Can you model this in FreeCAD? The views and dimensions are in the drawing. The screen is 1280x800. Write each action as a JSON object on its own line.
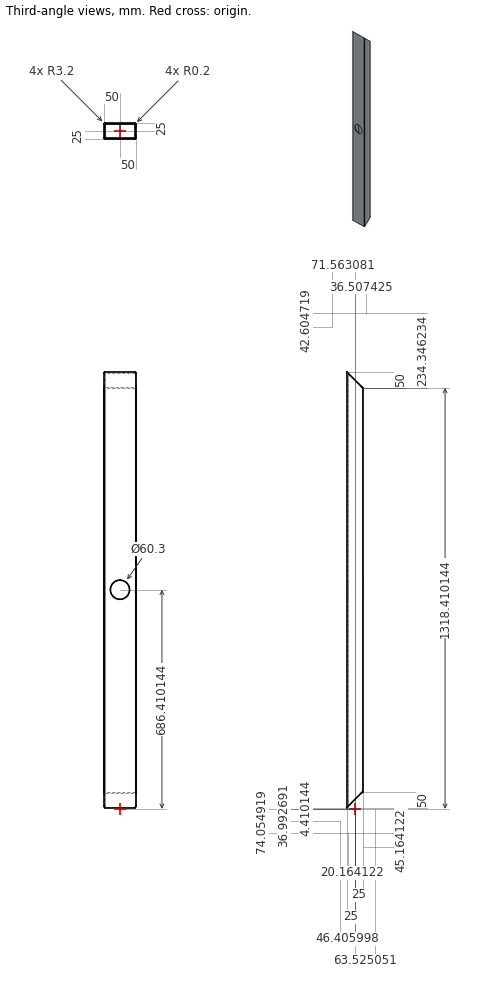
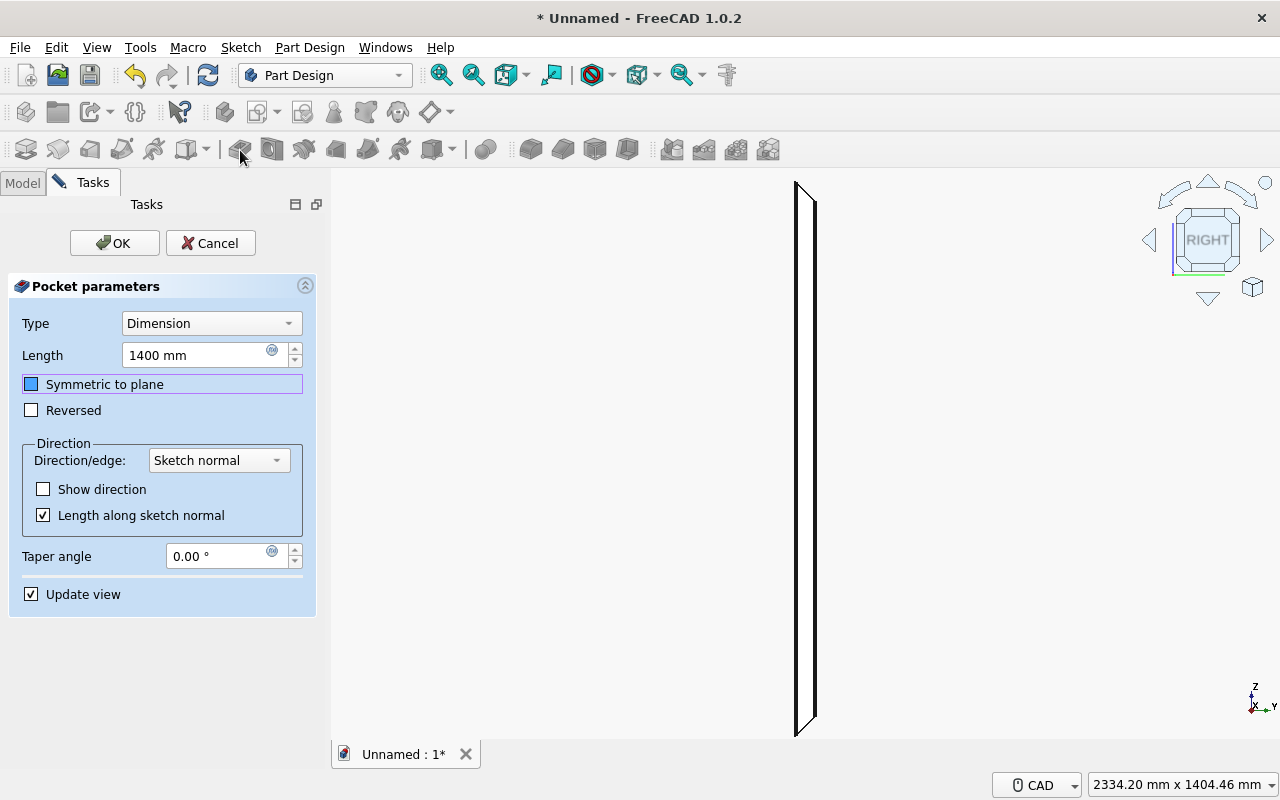
{"action": "left_click", "coordinate": [115, 243]}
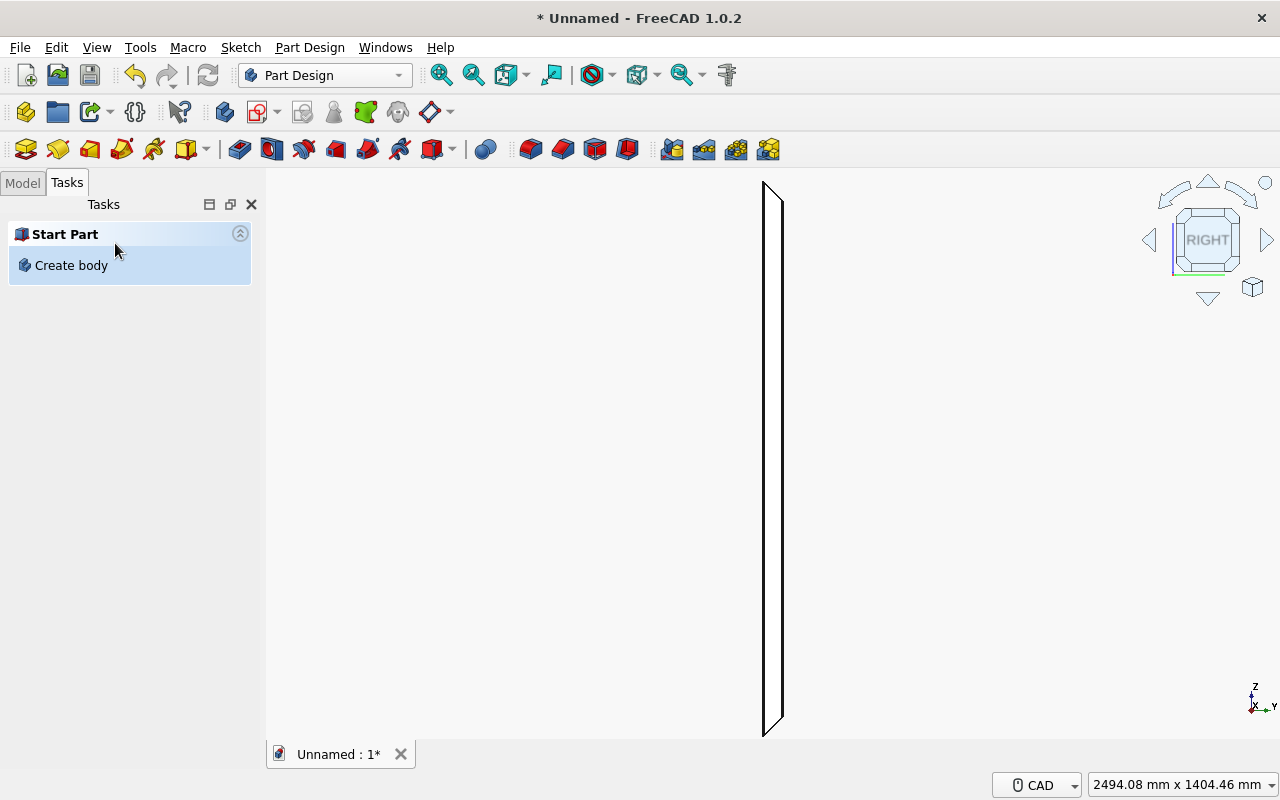
{"action": "key", "text": "4"}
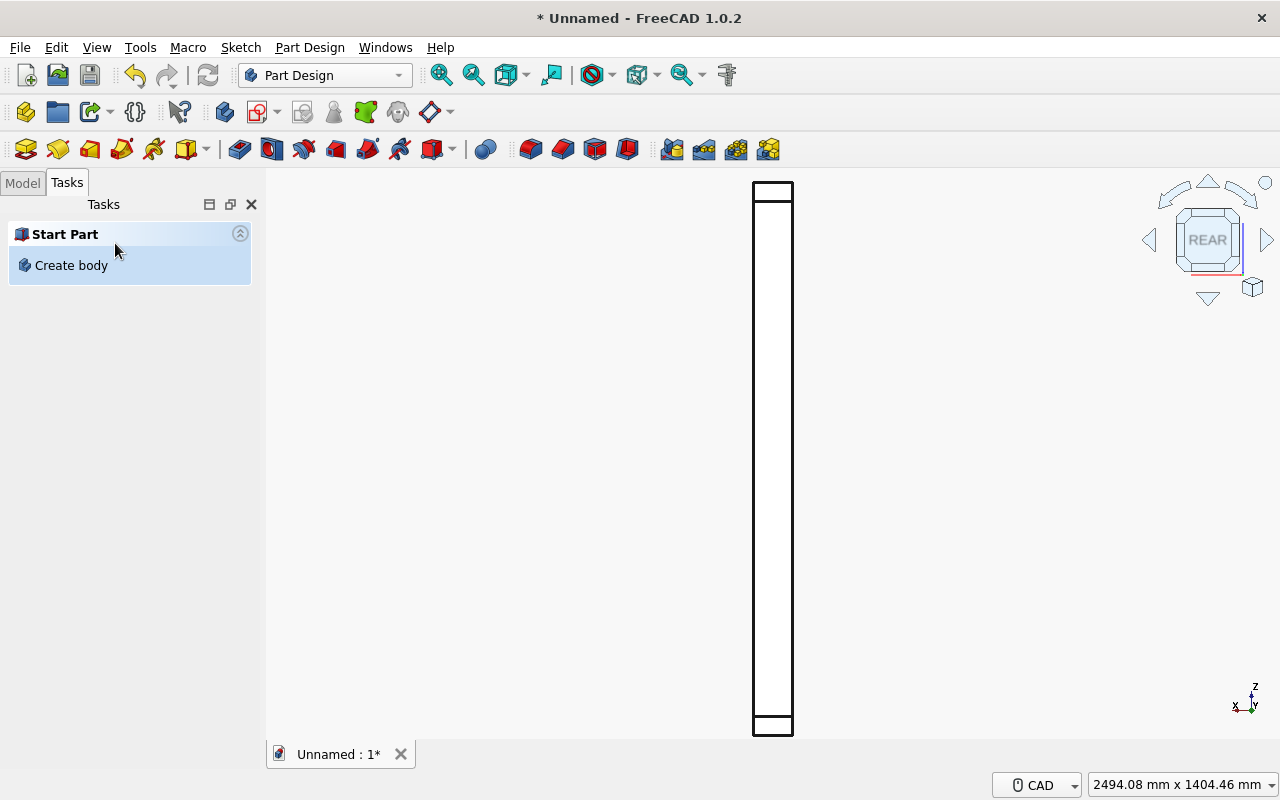
{"action": "left_click", "coordinate": [773, 238]}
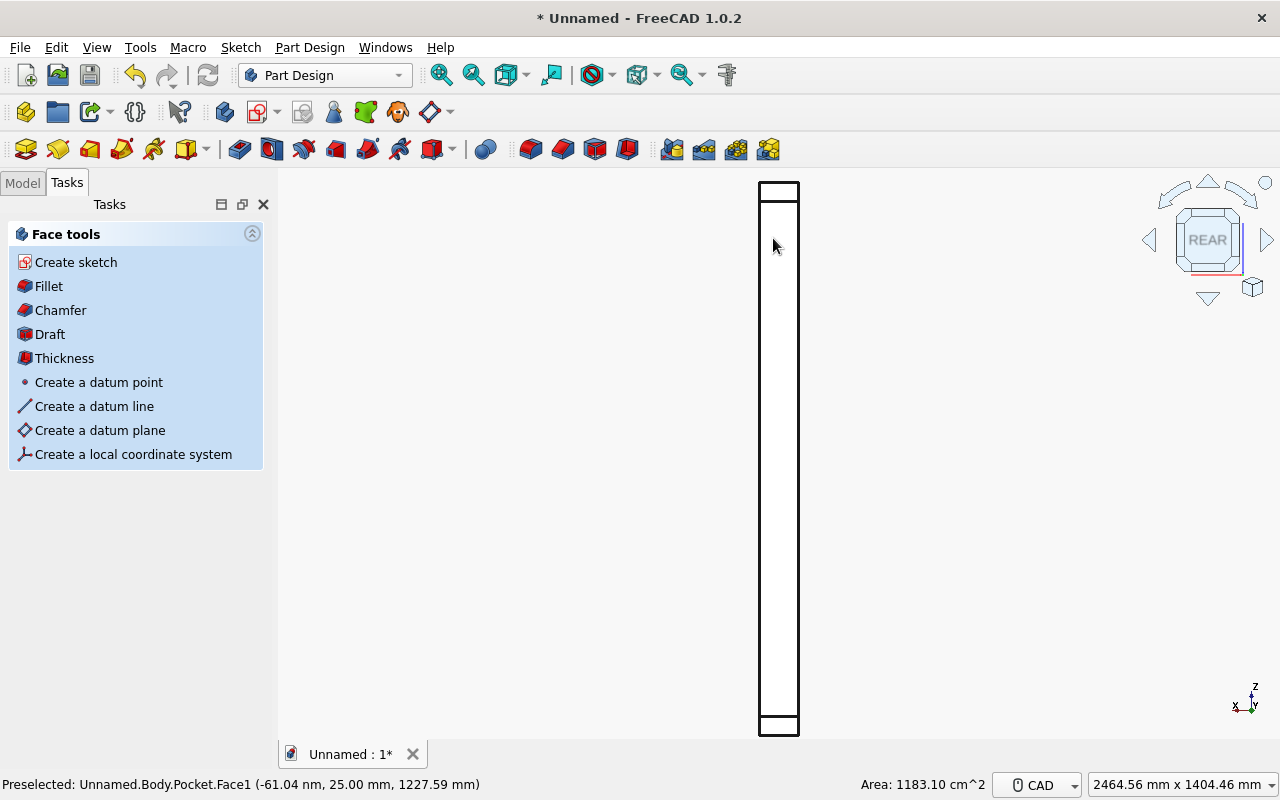
{"action": "left_click", "coordinate": [258, 112]}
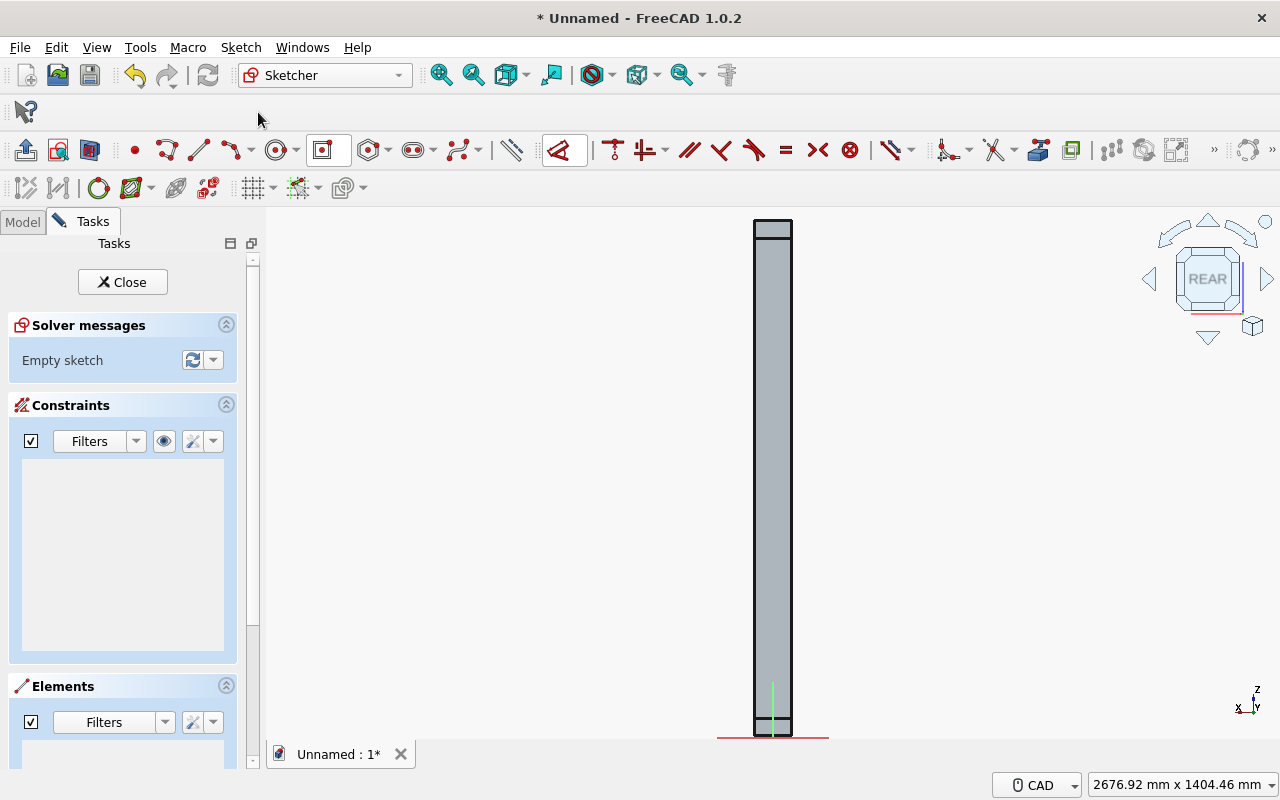
{"action": "scroll", "coordinate": [778, 479], "scroll_direction": "up", "scroll_amount": 13}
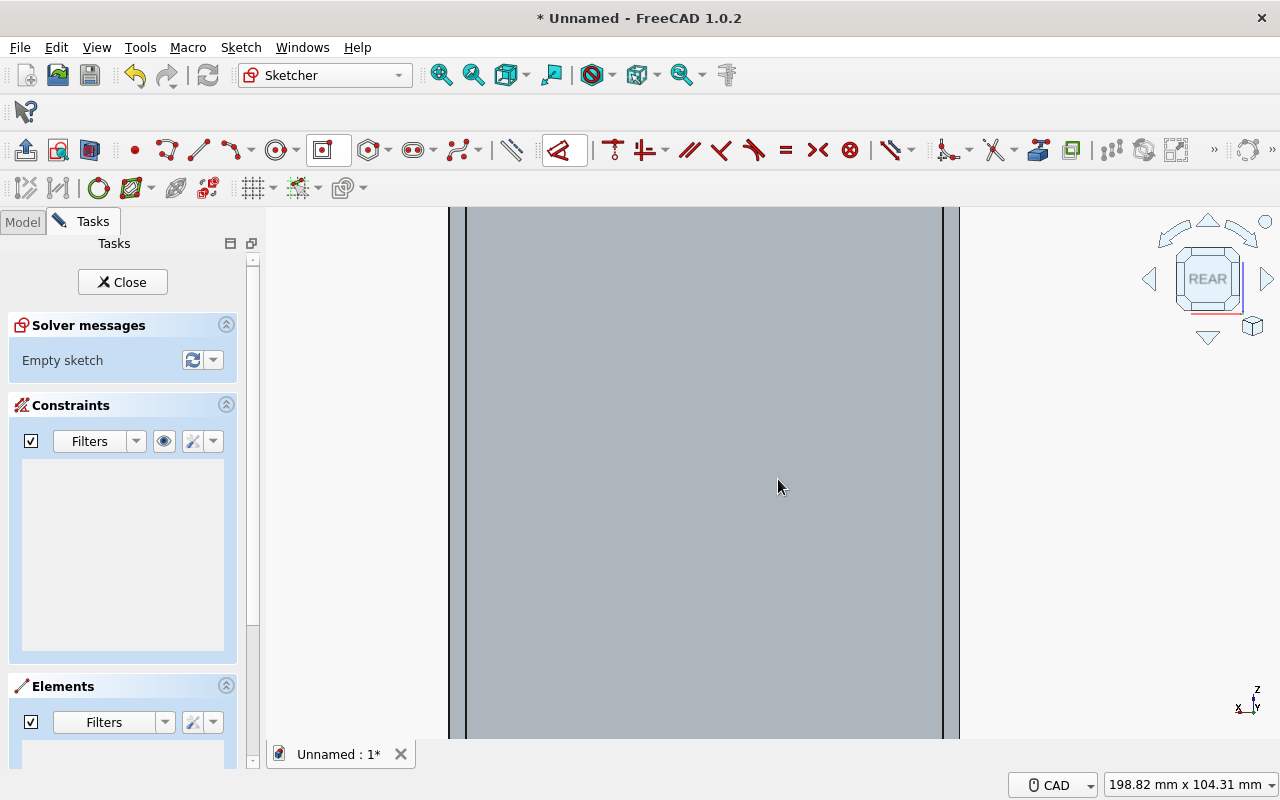
{"action": "key", "text": "g c"}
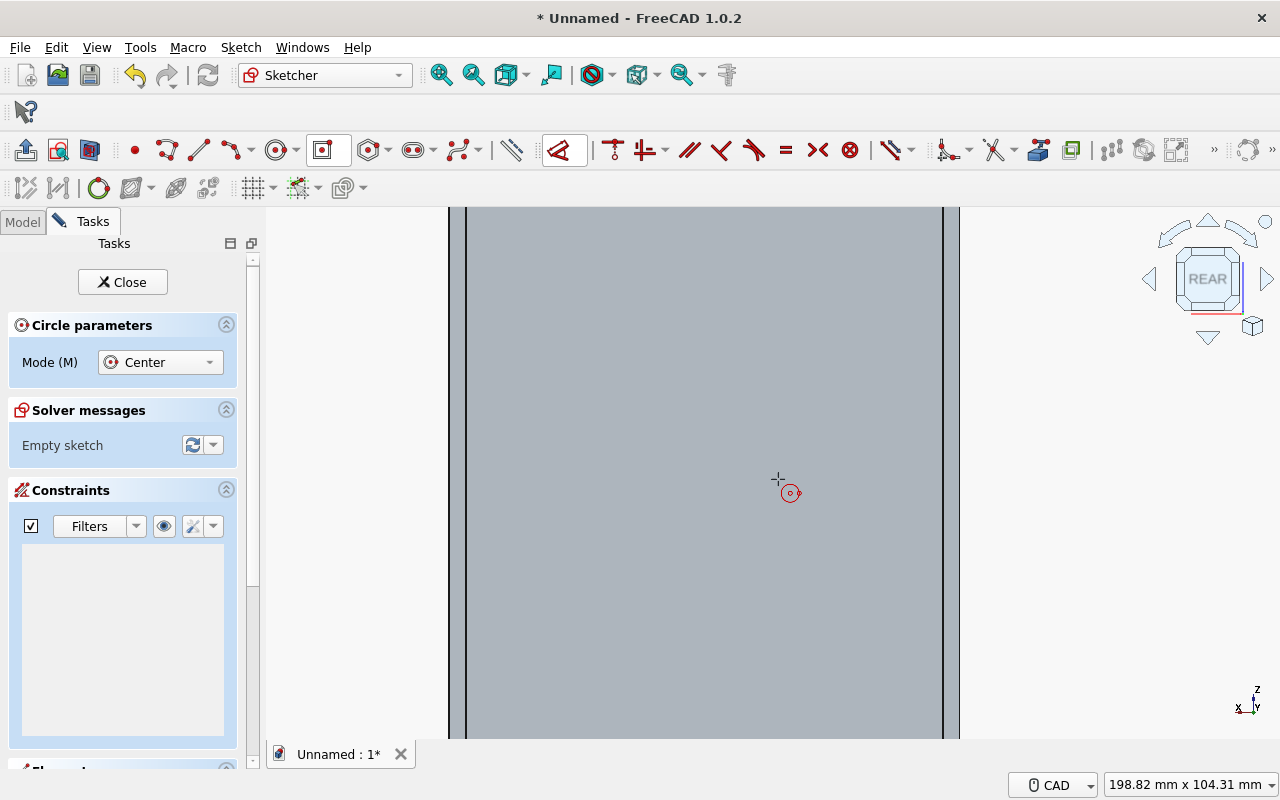
{"action": "left_click", "coordinate": [704, 461]}
{"action": "mouse_move", "coordinate": [813, 352]}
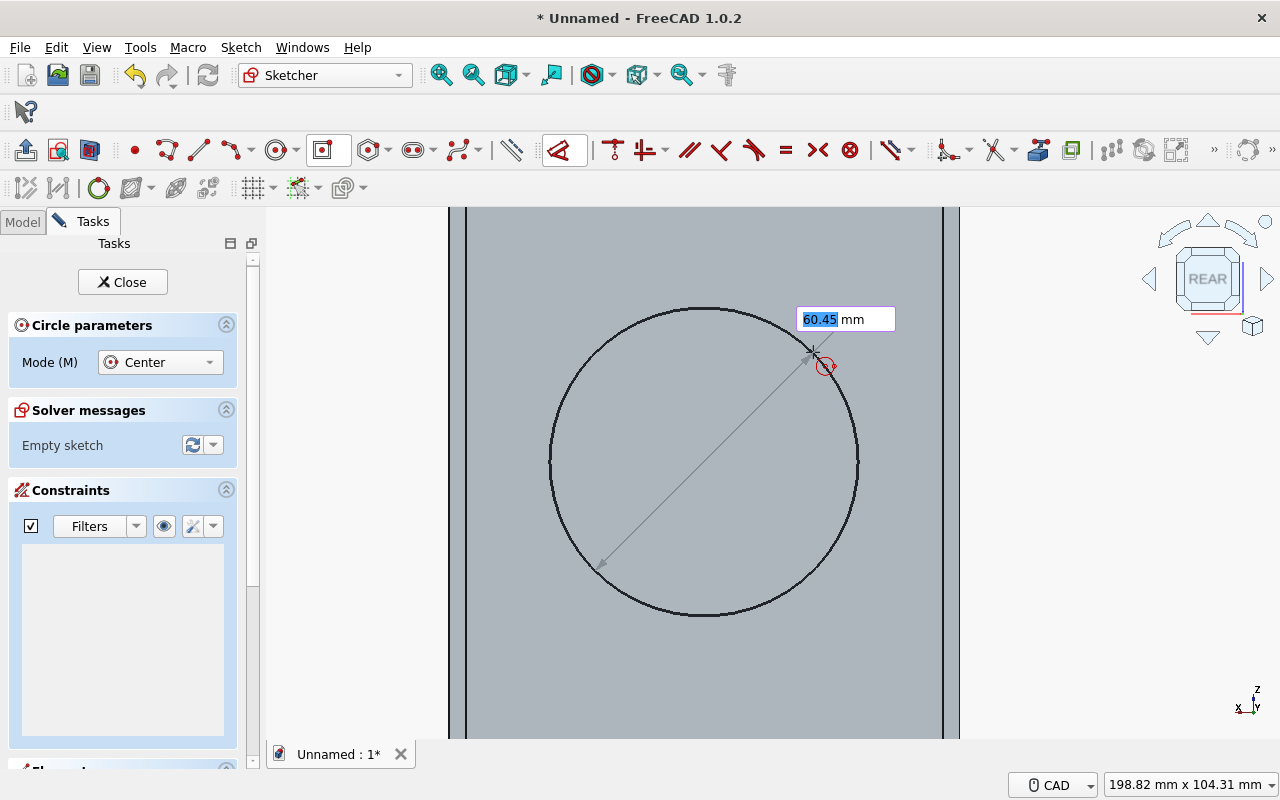
{"action": "type", "text": "60.3"}
{"action": "key", "text": "Return"}
{"action": "key", "text": "Escape"}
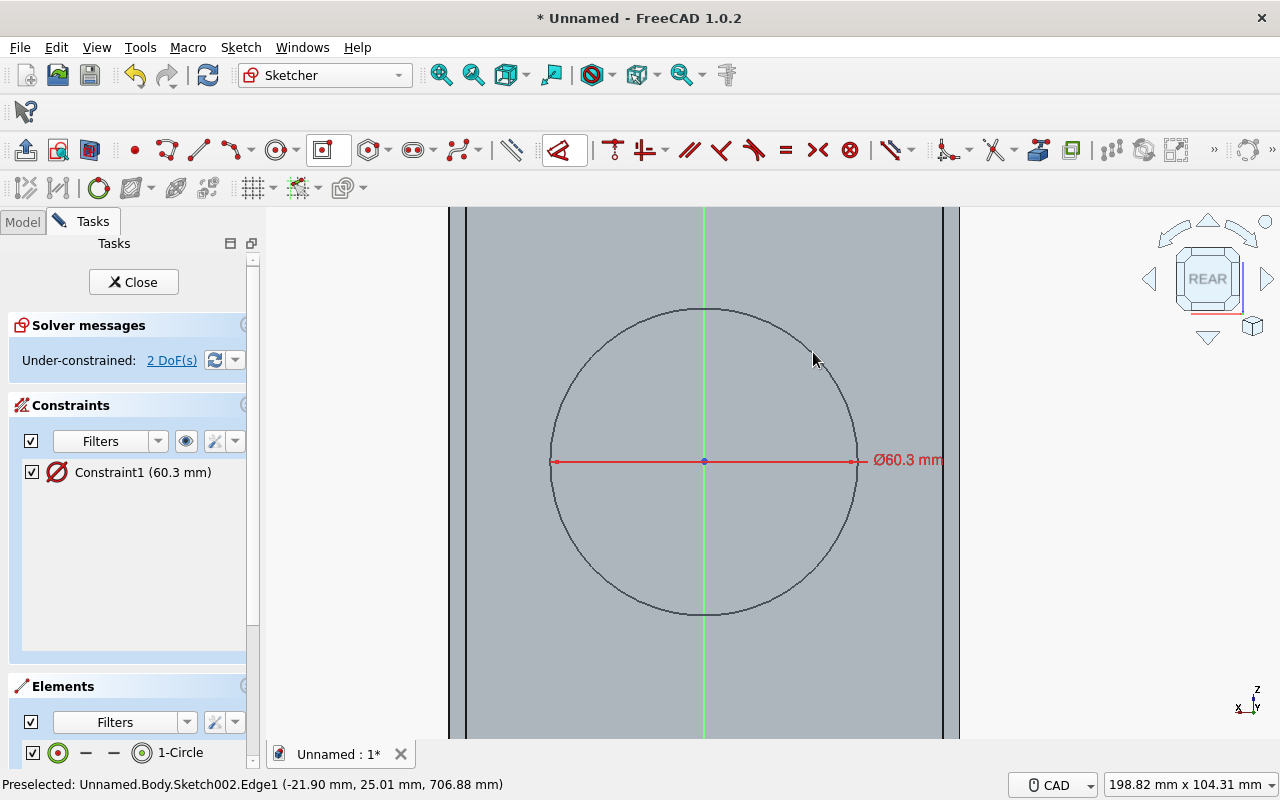
{"action": "left_click", "coordinate": [704, 462]}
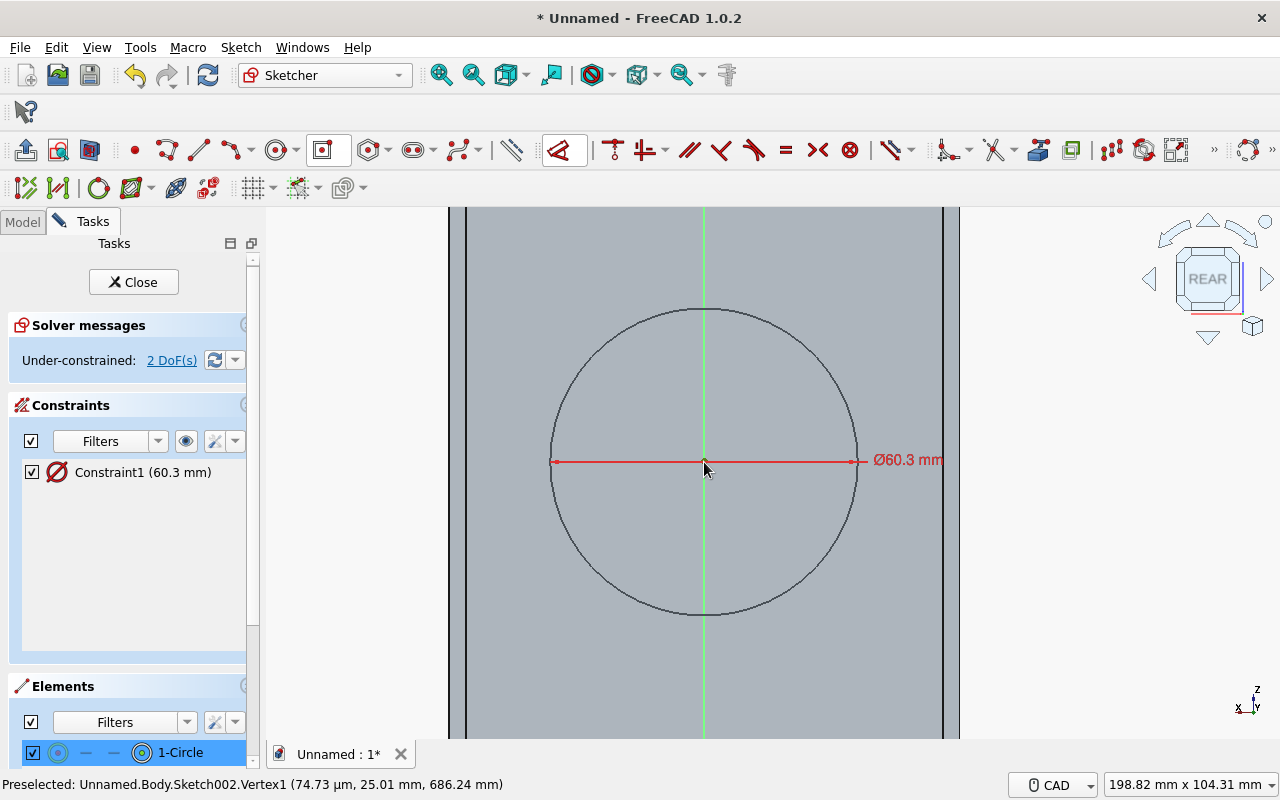
{"action": "left_click", "coordinate": [704, 677]}